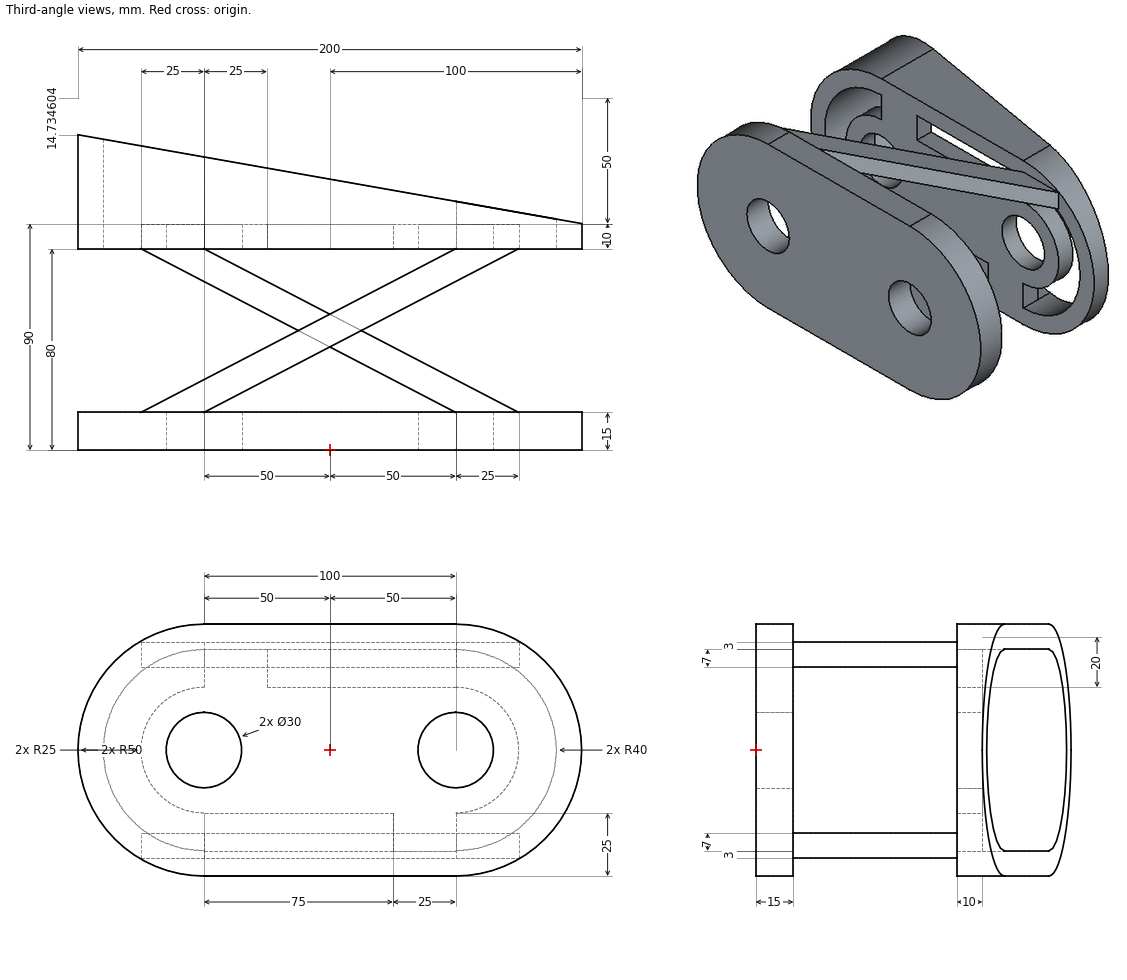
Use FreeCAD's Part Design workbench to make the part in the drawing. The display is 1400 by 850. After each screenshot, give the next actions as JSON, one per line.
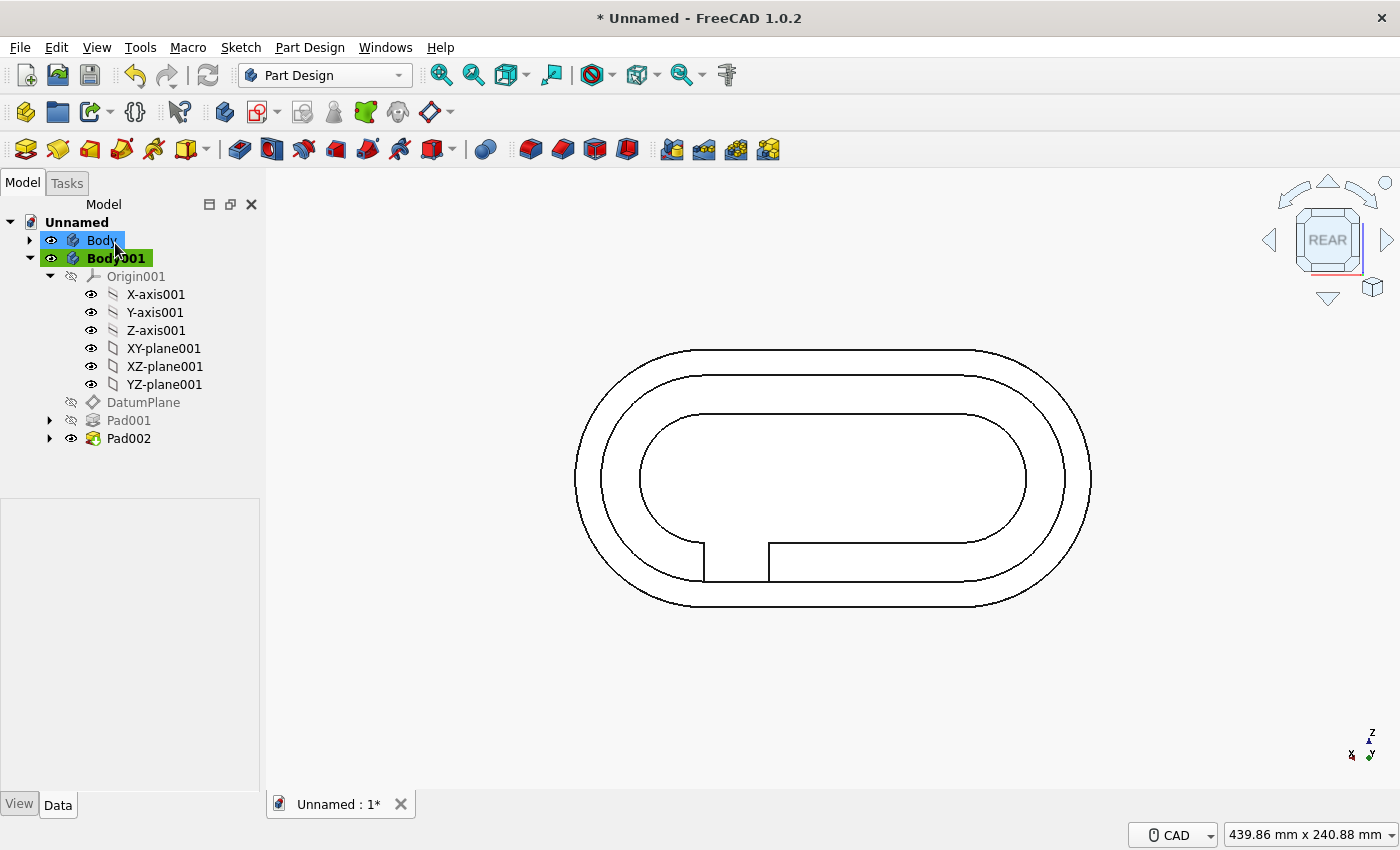
{"action": "key", "text": "0"}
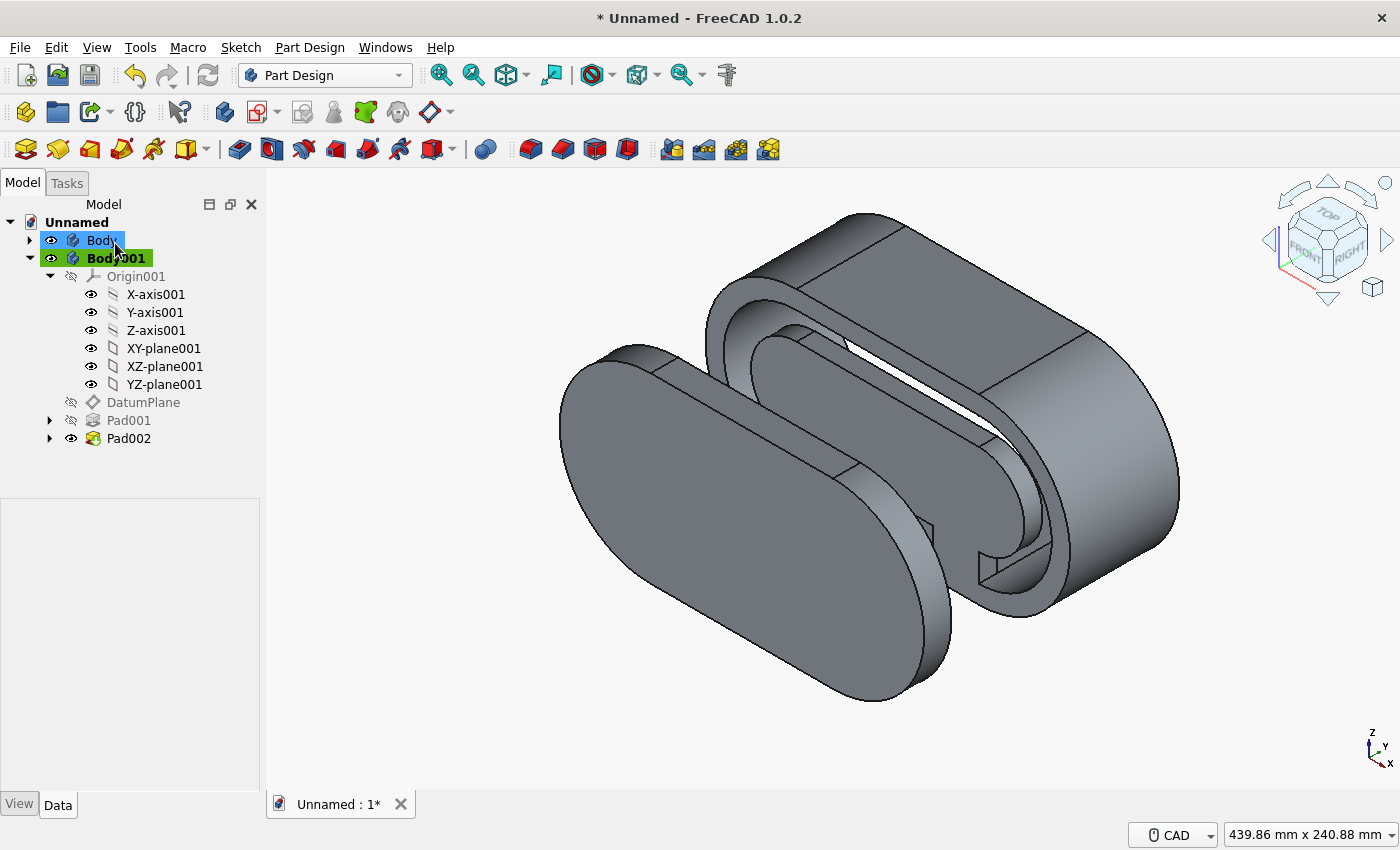
{"action": "left_click", "coordinate": [968, 324]}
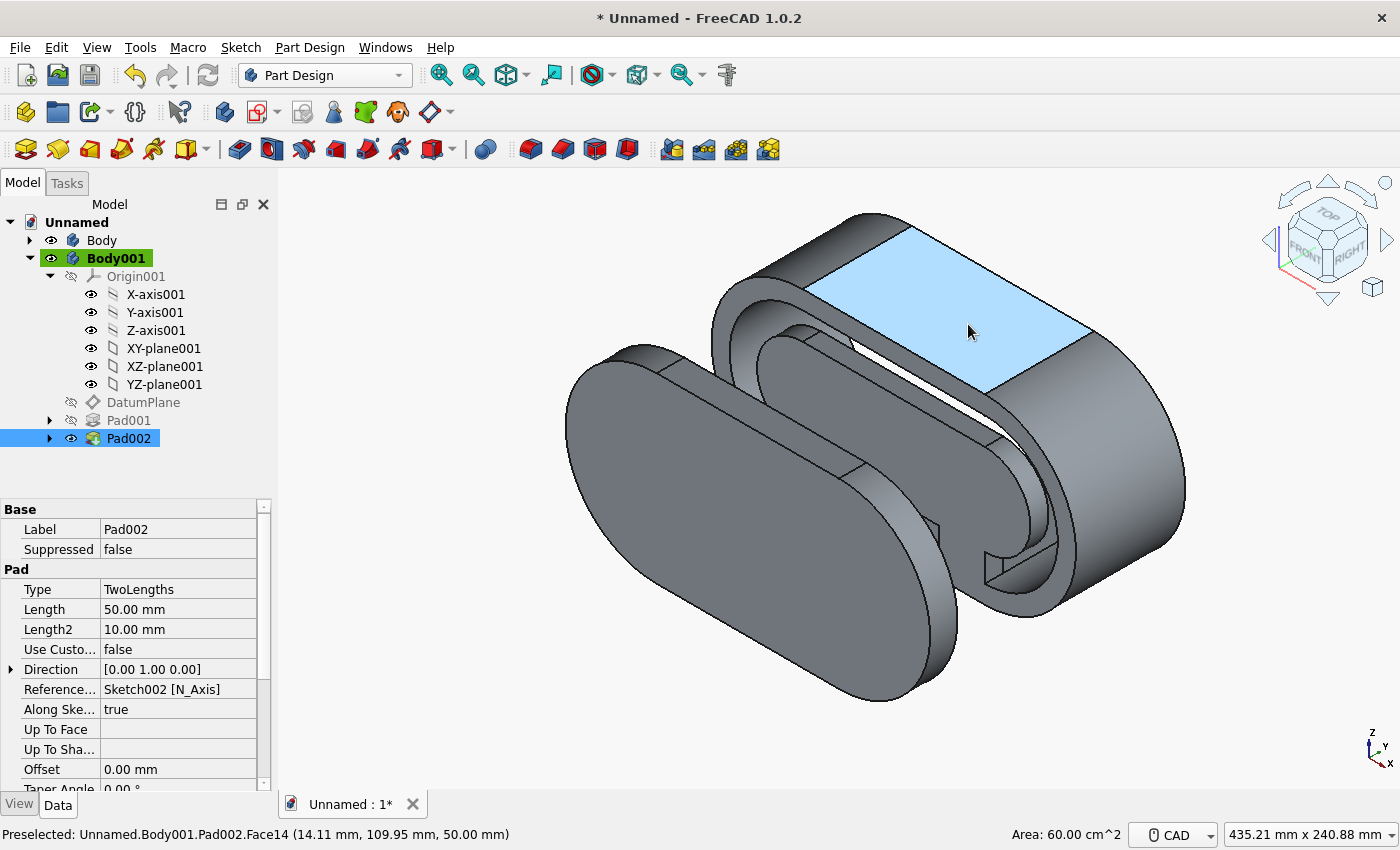
{"action": "left_click", "coordinate": [258, 112]}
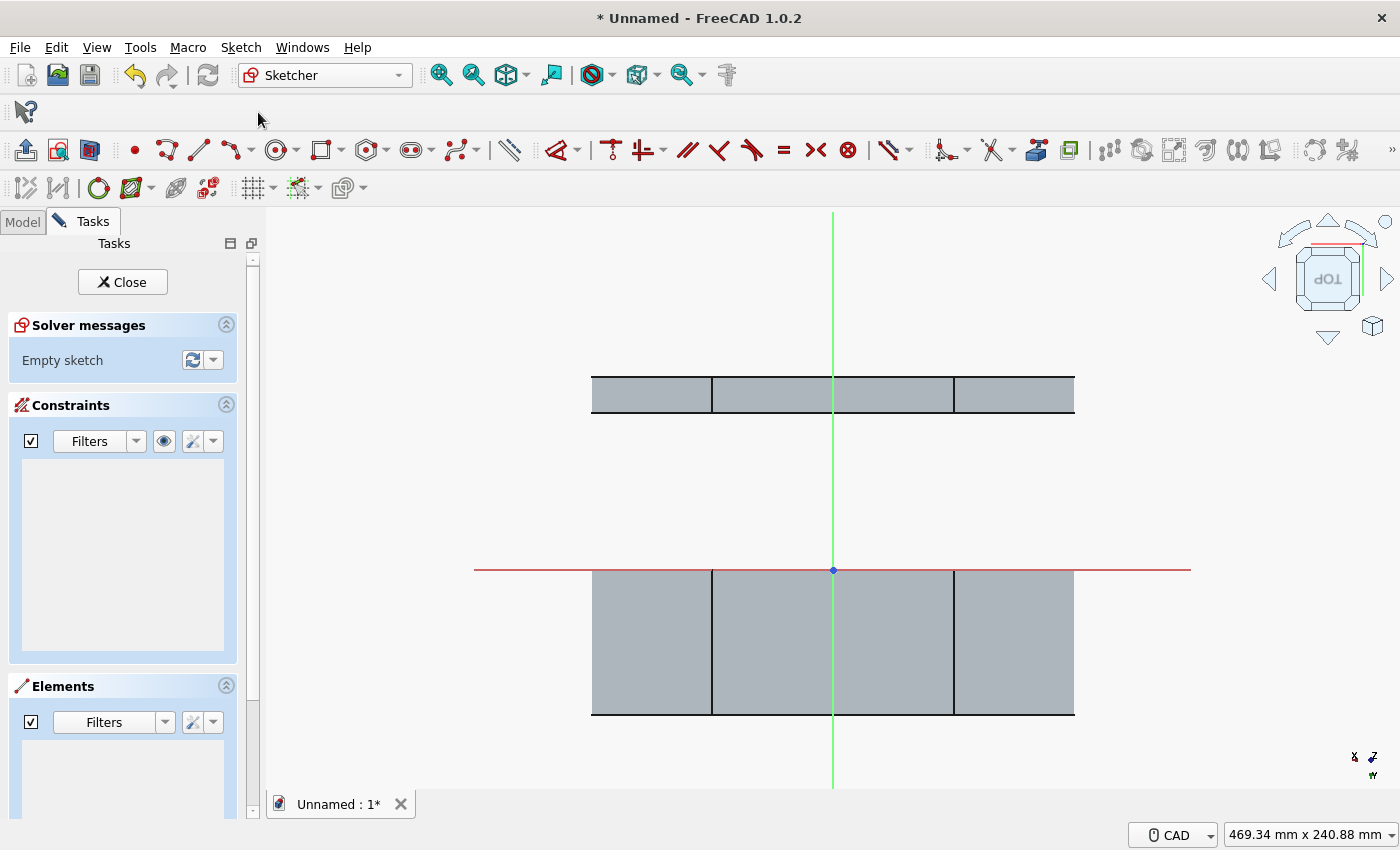
{"action": "scroll", "coordinate": [972, 761], "scroll_direction": "up", "scroll_amount": 2}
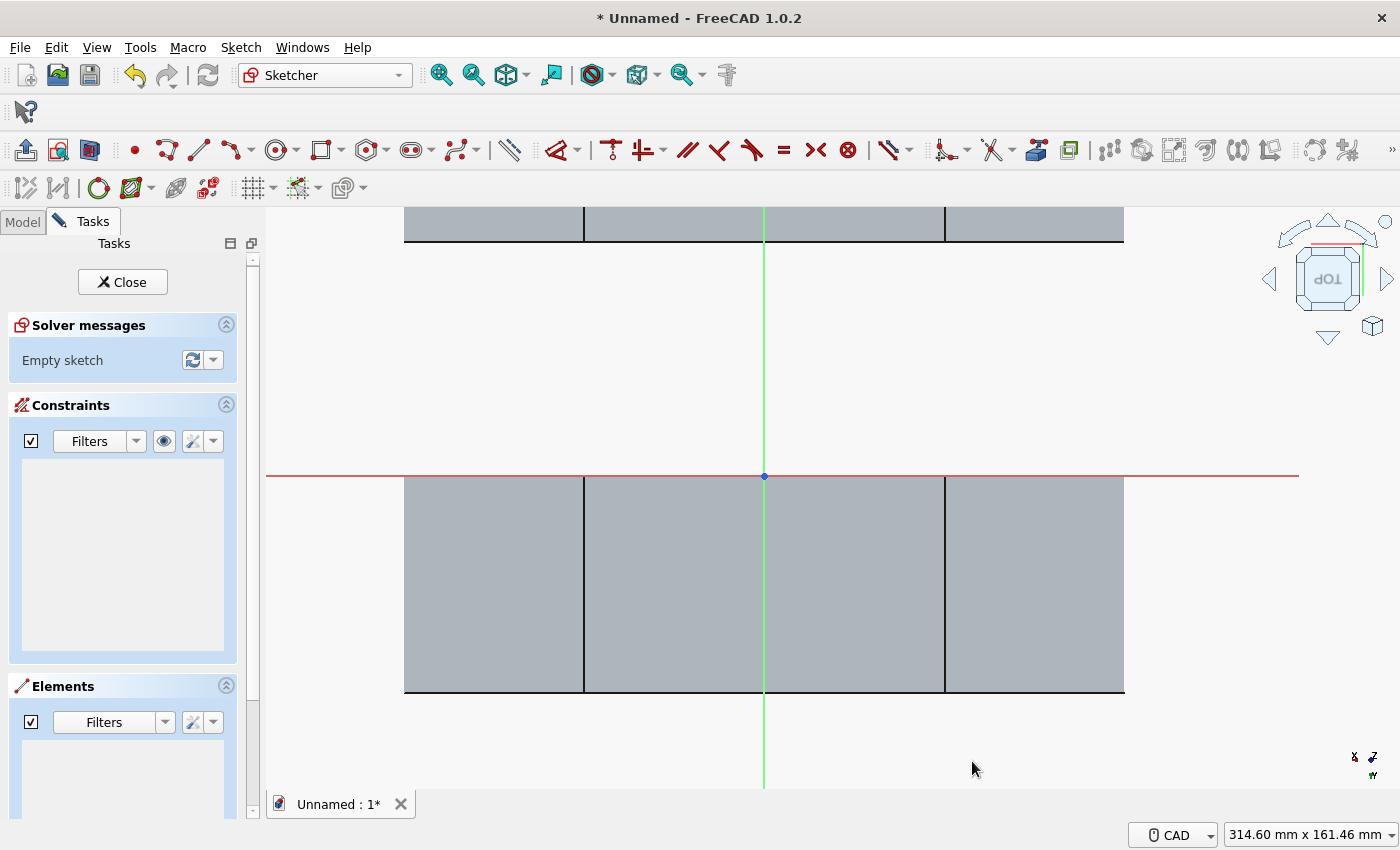
{"action": "left_click", "coordinate": [168, 150]}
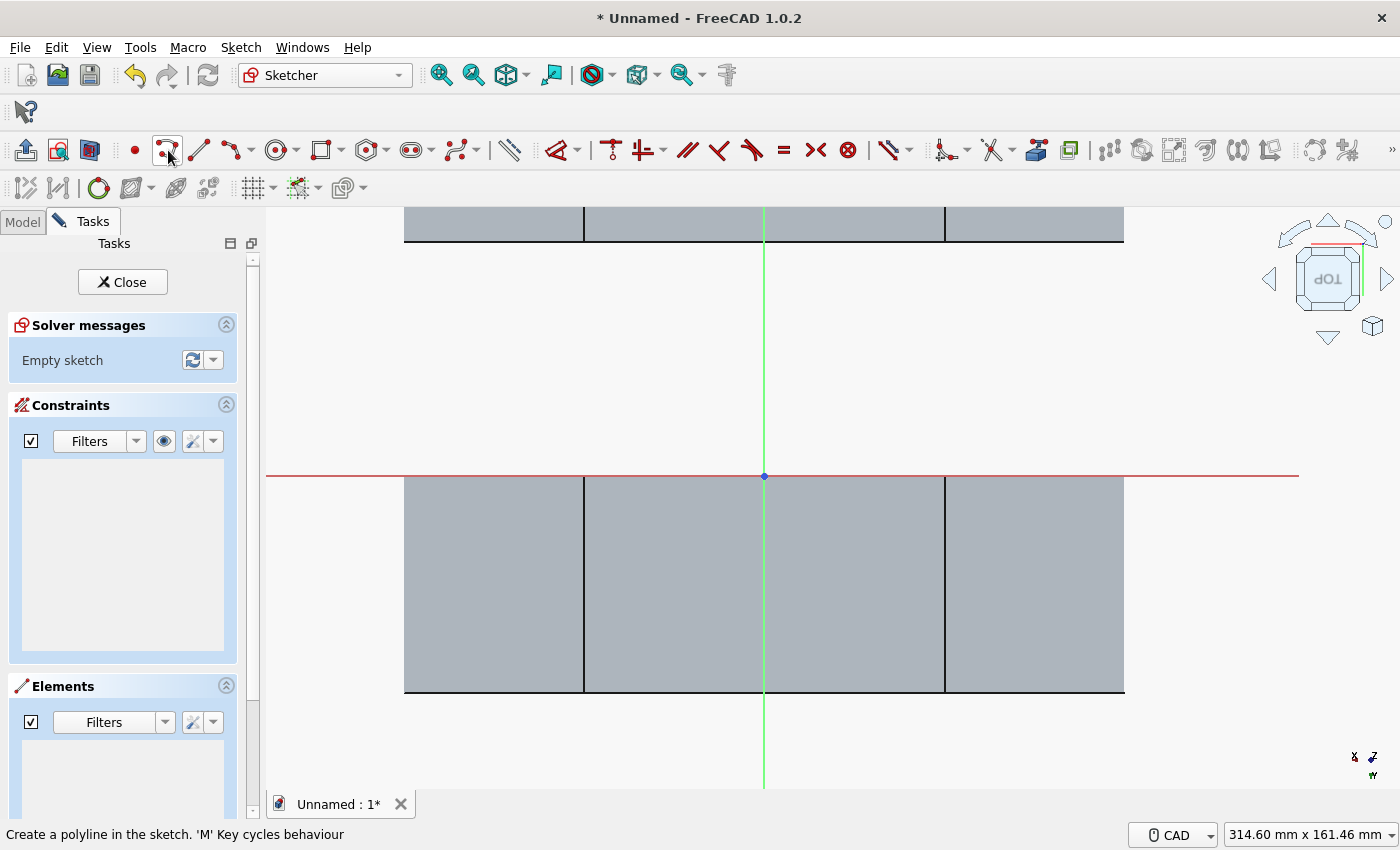
{"action": "left_click", "coordinate": [404, 512]}
{"action": "left_click", "coordinate": [404, 693]}
{"action": "left_click", "coordinate": [1125, 693]}
{"action": "left_click", "coordinate": [1125, 639]}
{"action": "left_click", "coordinate": [404, 513]}
{"action": "key", "text": "Escape"}
{"action": "key", "text": "Escape"}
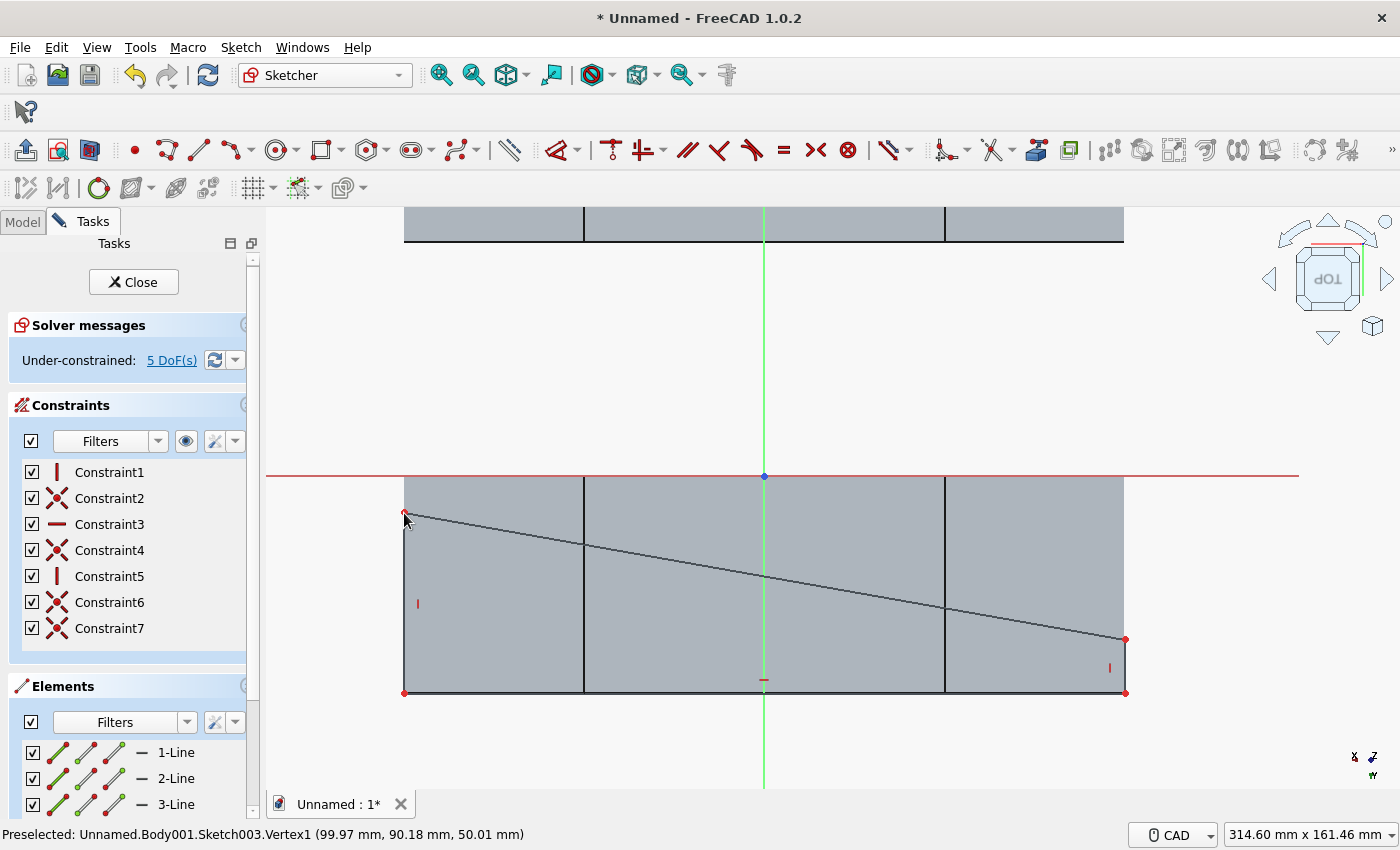
{"action": "left_click", "coordinate": [556, 150]}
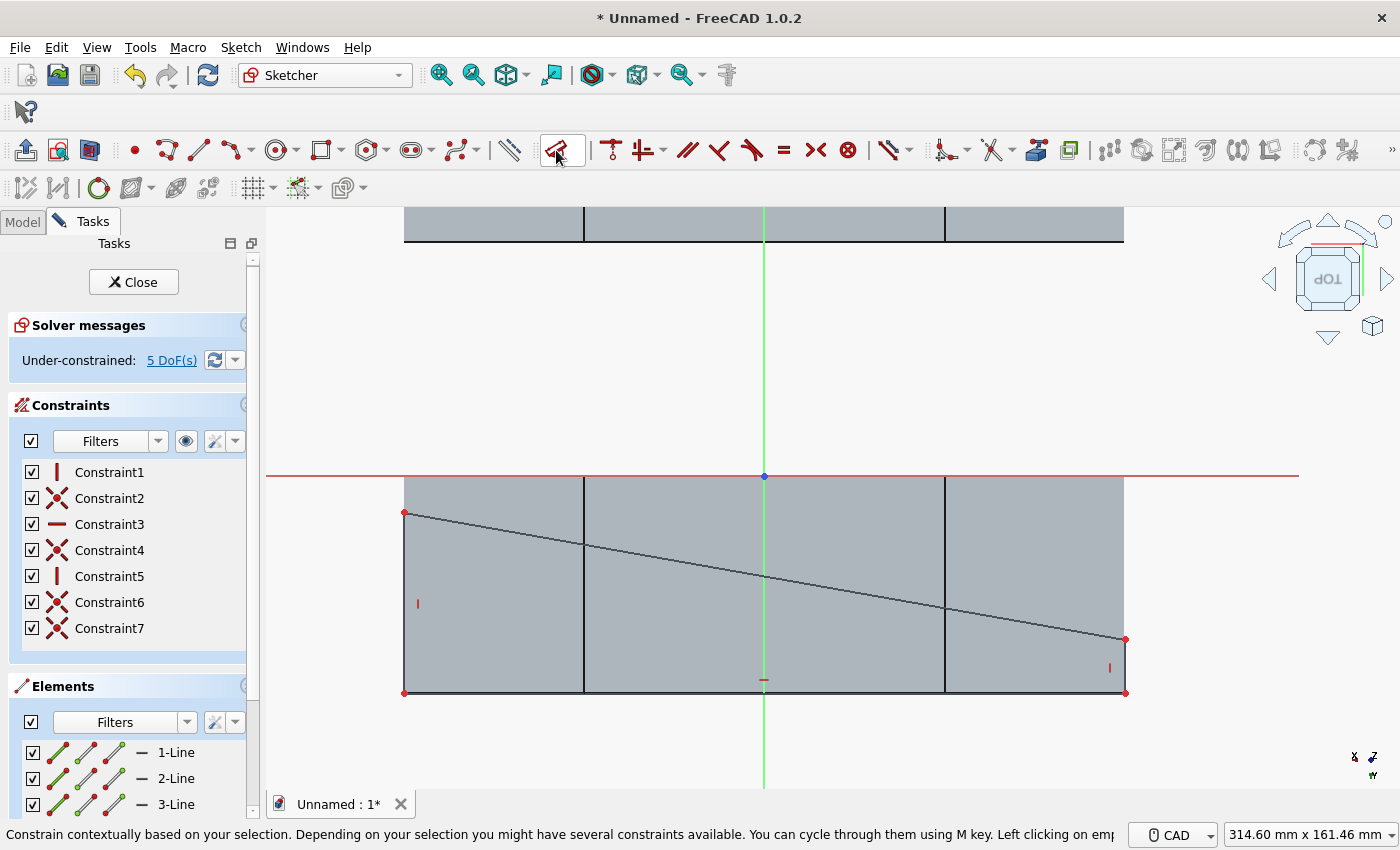
{"action": "left_click", "coordinate": [404, 567]}
{"action": "left_click", "coordinate": [370, 604]}